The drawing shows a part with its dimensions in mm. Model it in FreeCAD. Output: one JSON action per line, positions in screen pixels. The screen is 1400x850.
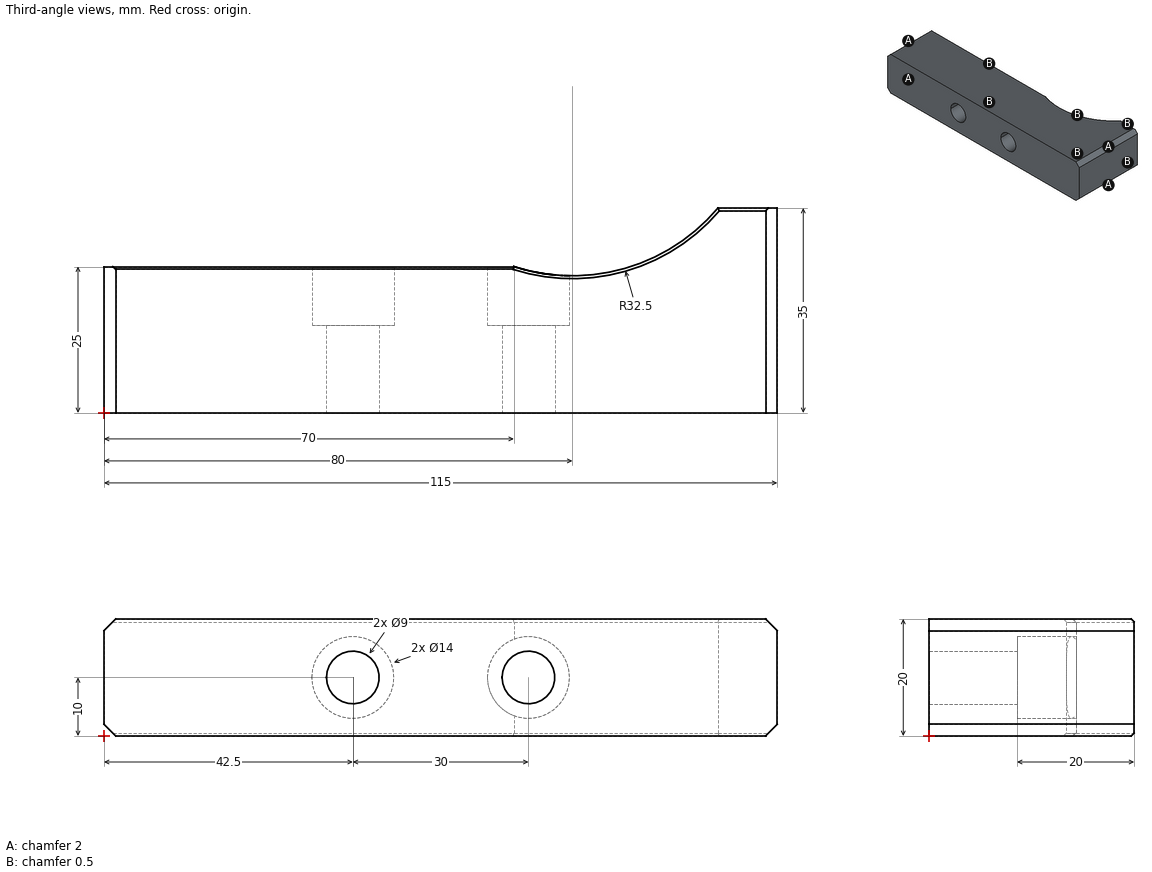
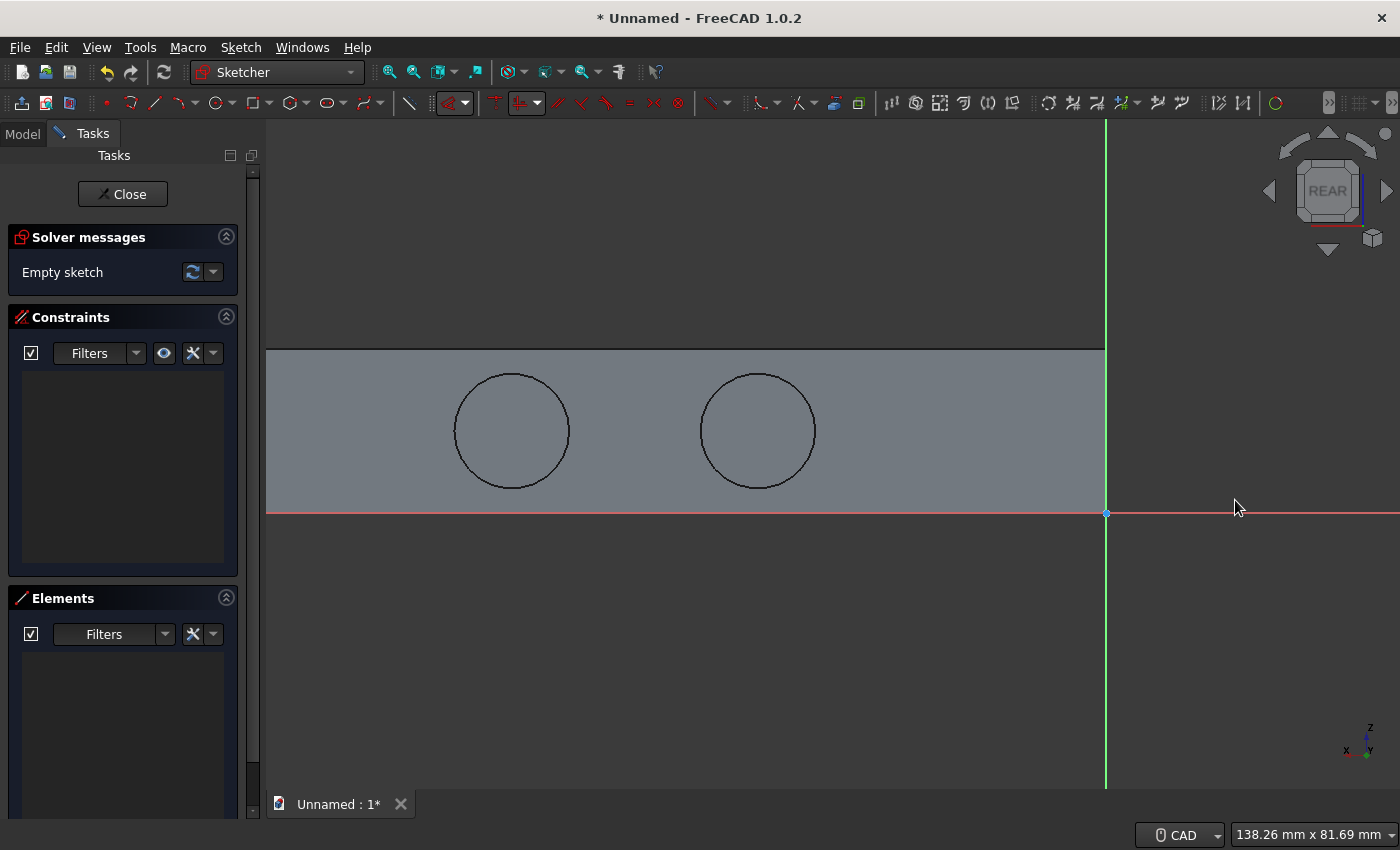
{"action": "left_click", "coordinate": [216, 104]}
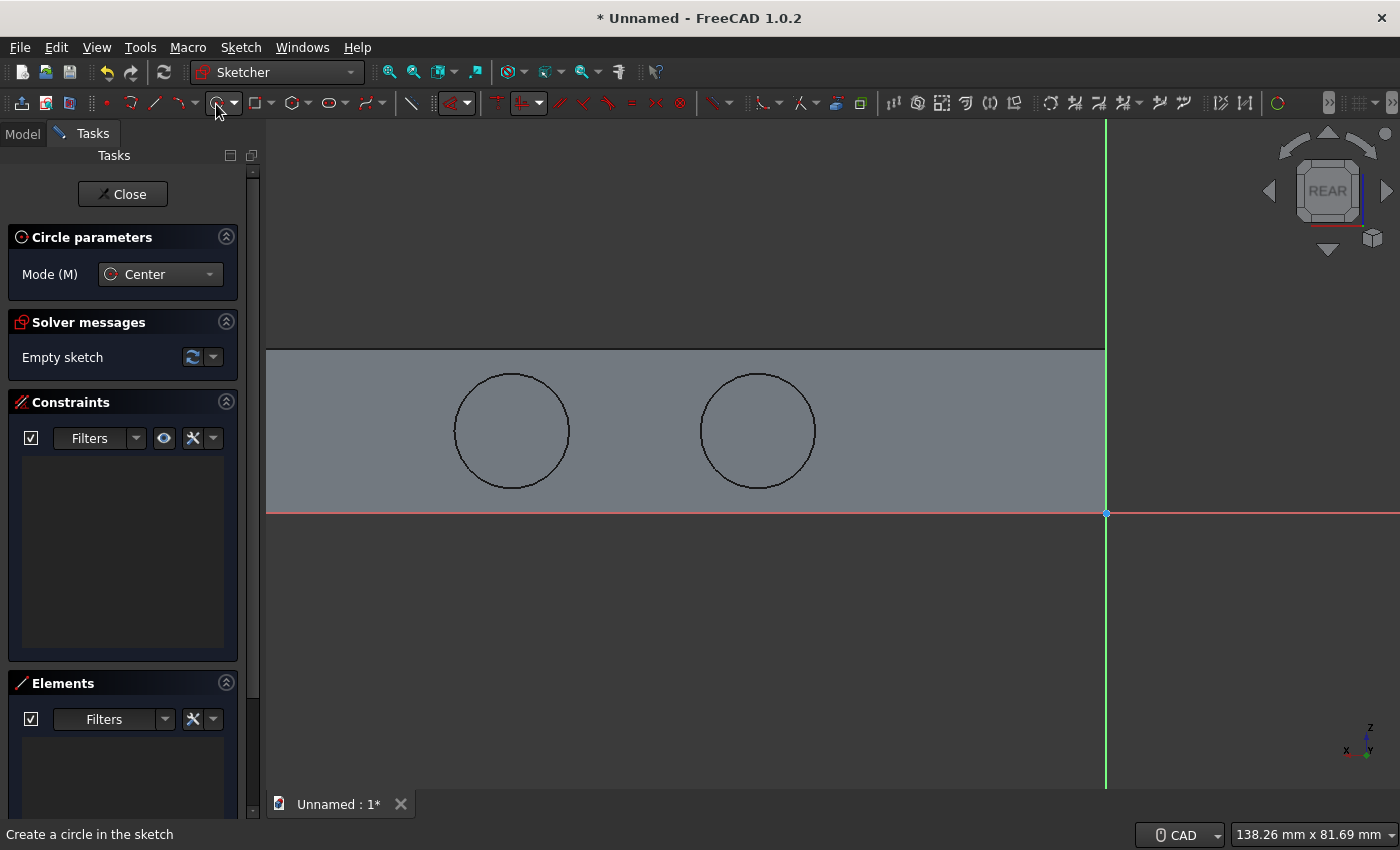
{"action": "left_click", "coordinate": [758, 431]}
{"action": "left_click", "coordinate": [784, 405]}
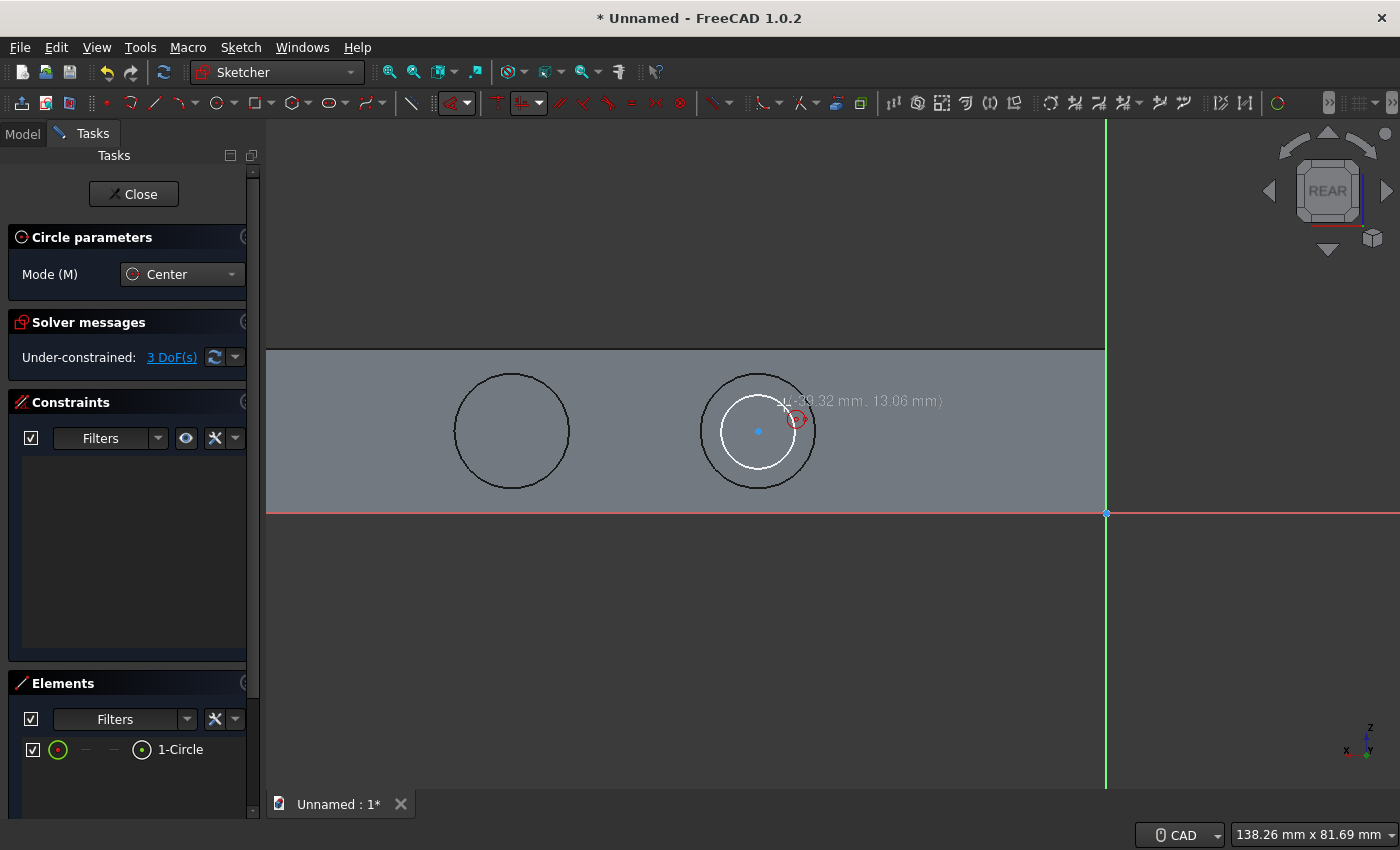
{"action": "left_click", "coordinate": [512, 431]}
{"action": "left_click", "coordinate": [538, 405]}
{"action": "key", "text": "Escape"}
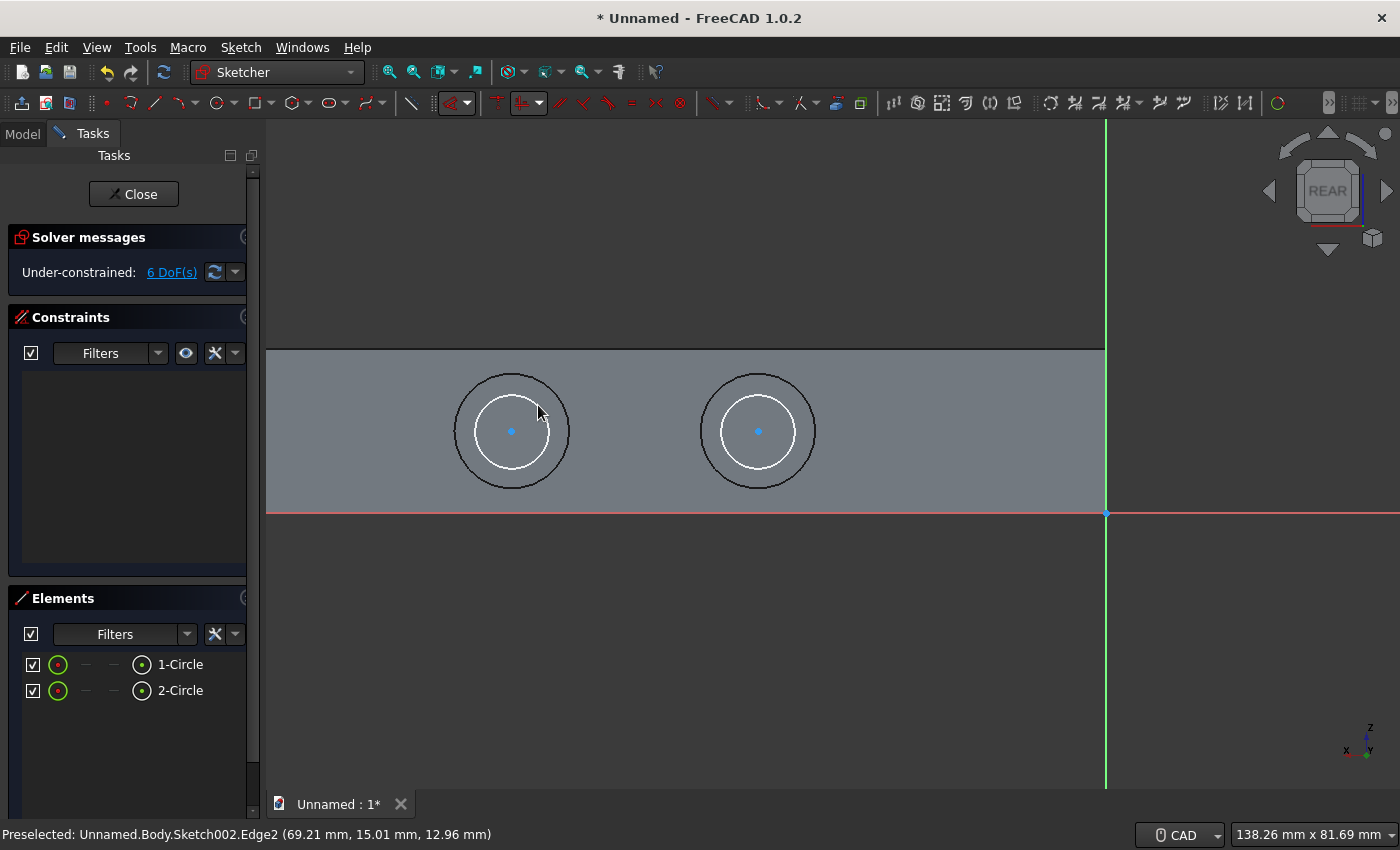
{"action": "left_click", "coordinate": [784, 406]}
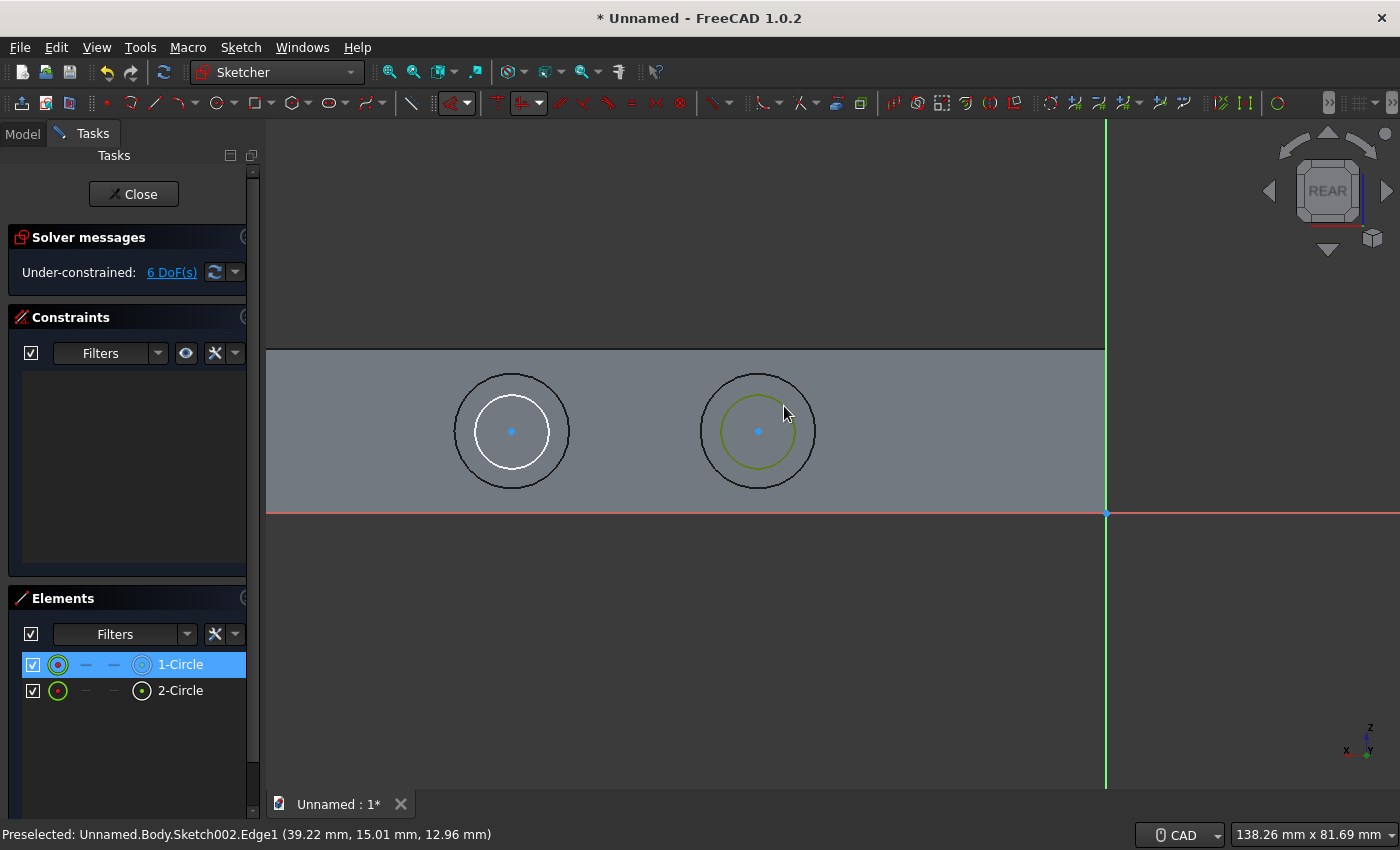
{"action": "left_click", "coordinate": [538, 406]}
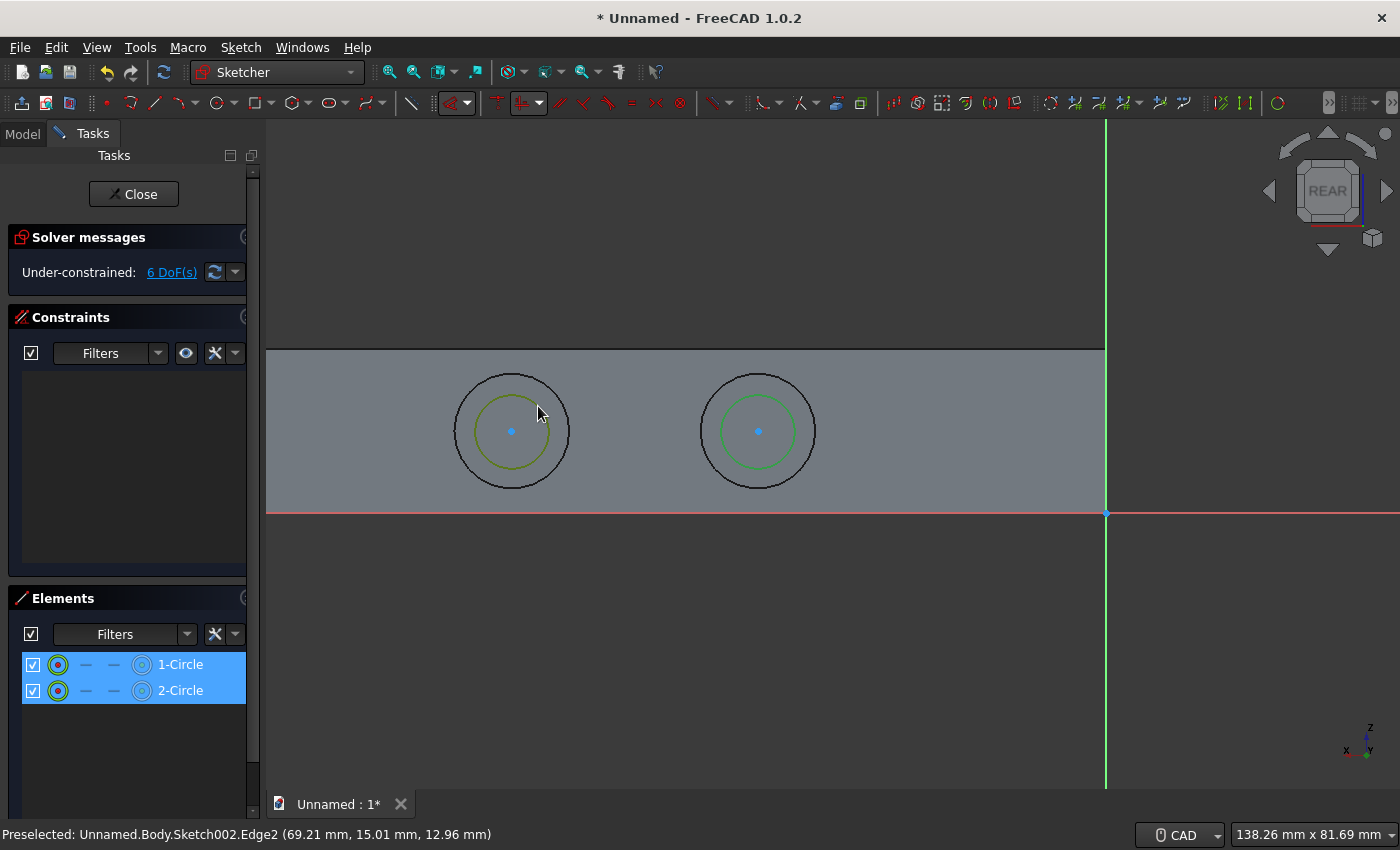
{"action": "left_click", "coordinate": [632, 104]}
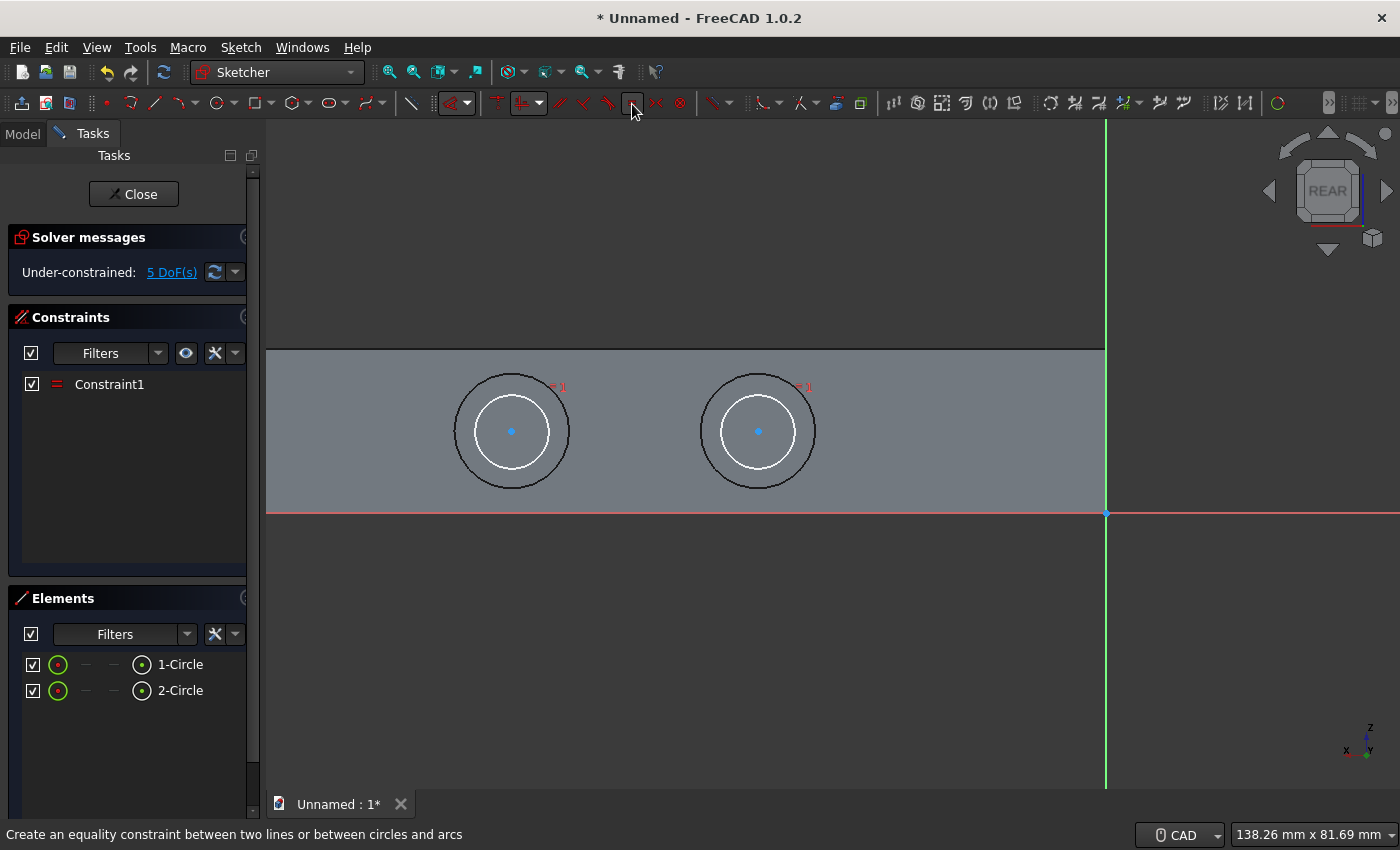
{"action": "left_click", "coordinate": [758, 432]}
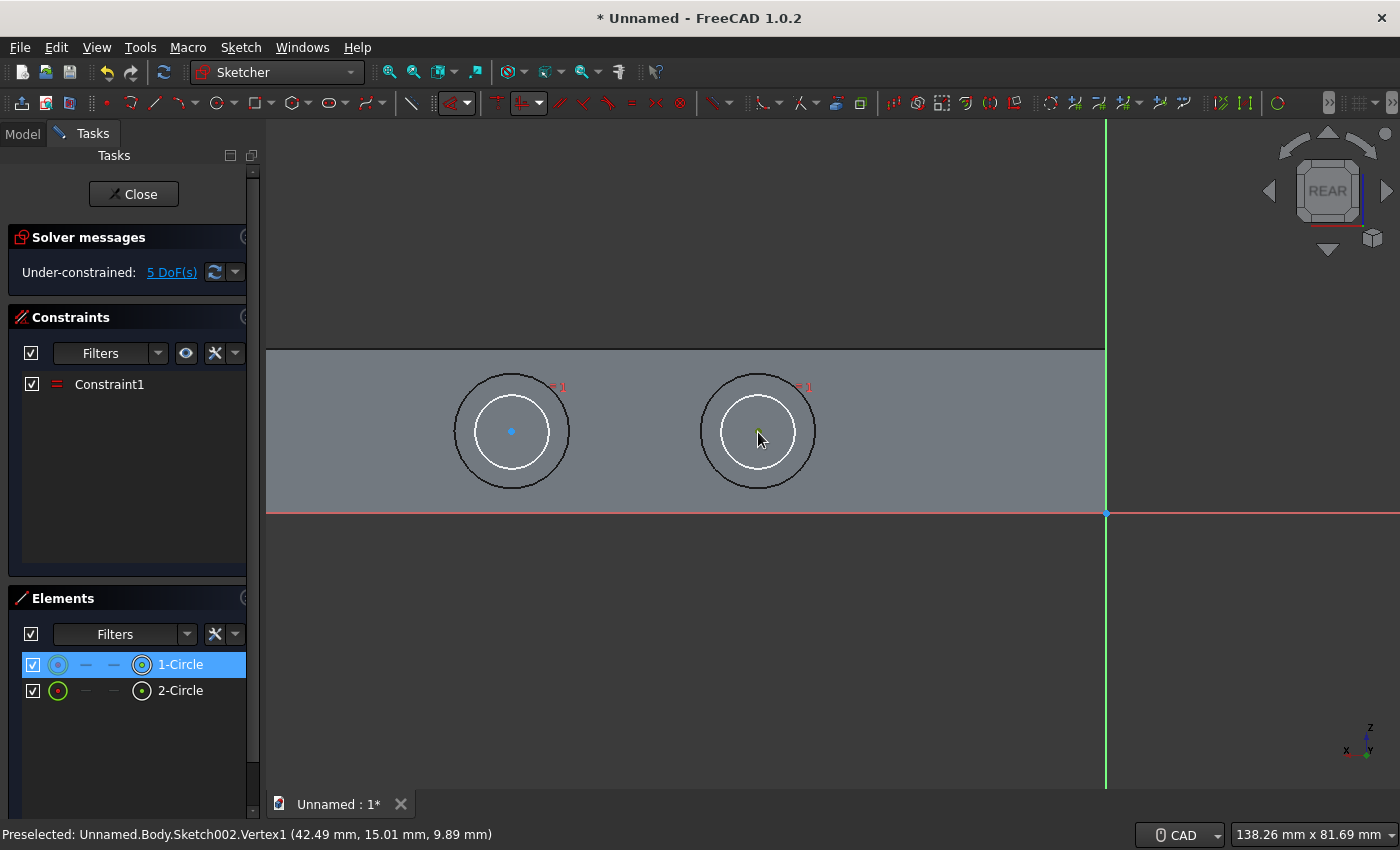
{"action": "left_click", "coordinate": [512, 432]}